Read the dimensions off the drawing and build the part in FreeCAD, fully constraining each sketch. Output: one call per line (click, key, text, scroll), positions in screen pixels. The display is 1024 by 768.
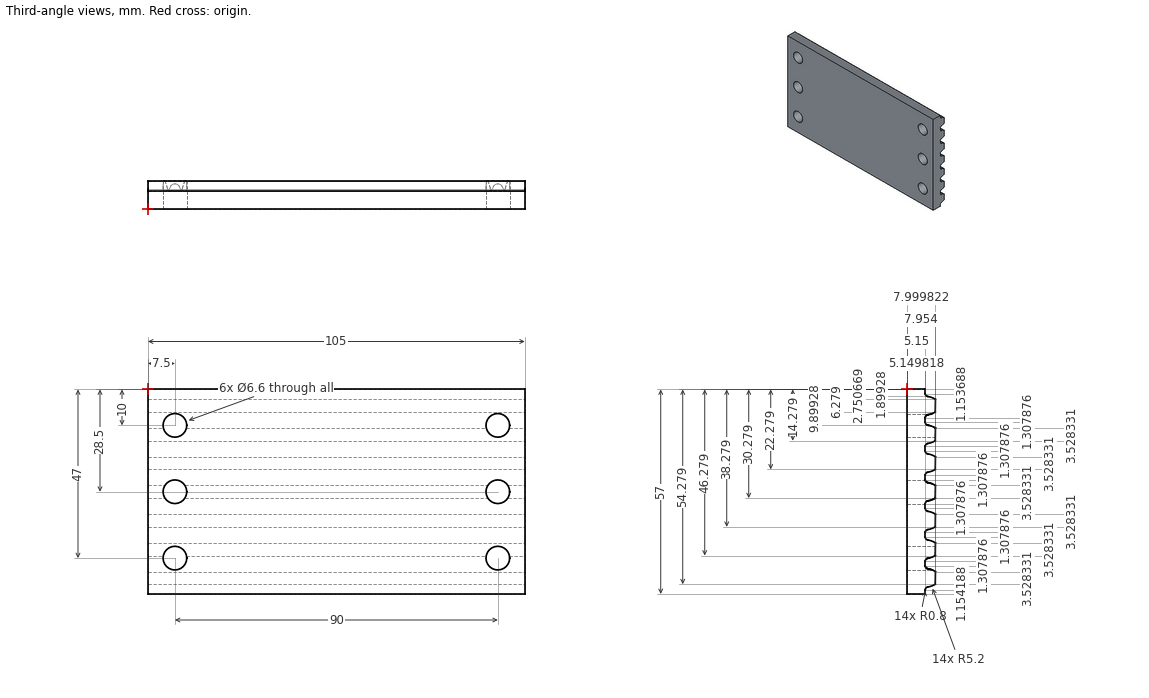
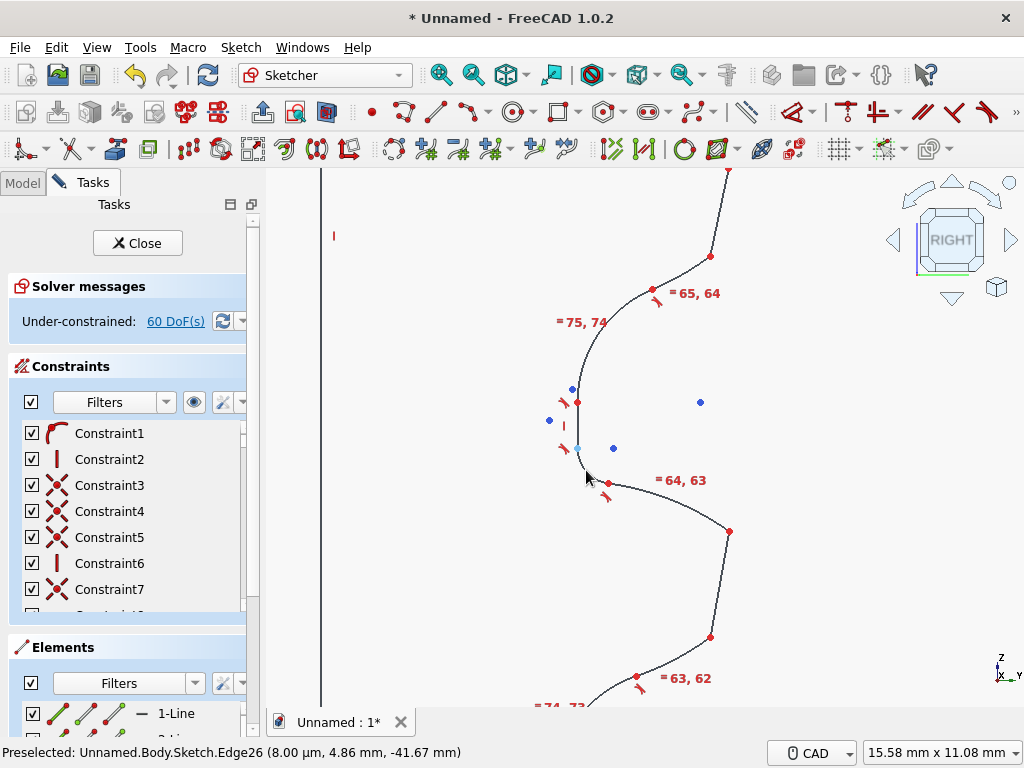
click(581, 463)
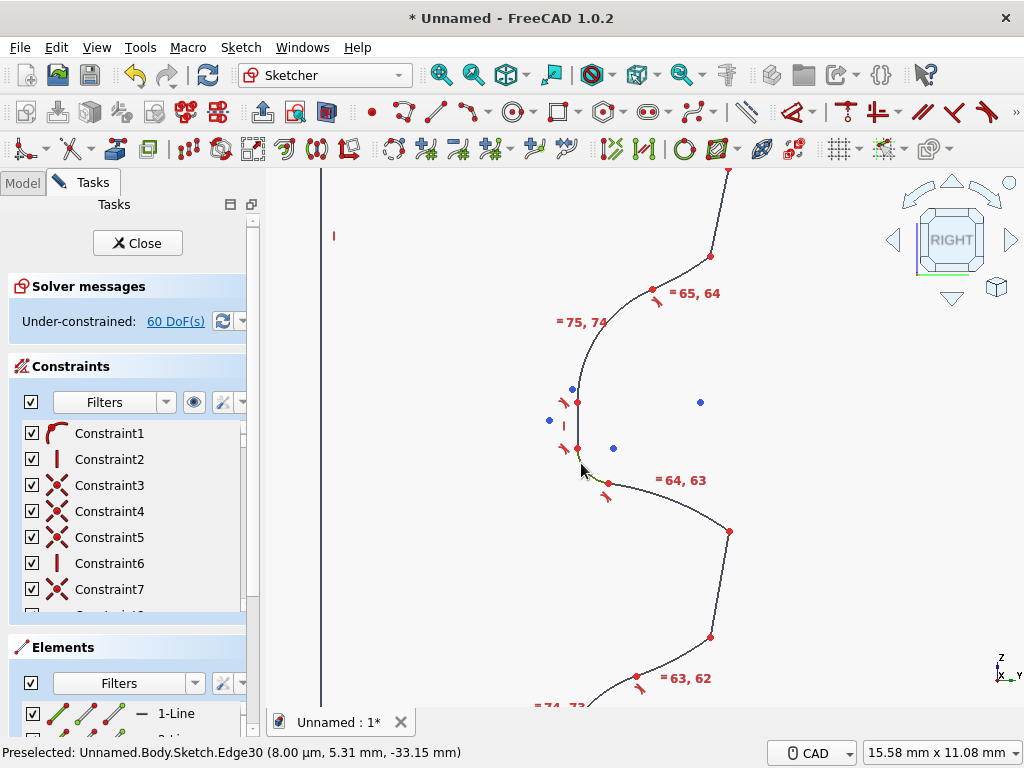
scroll(586, 469, down, 10)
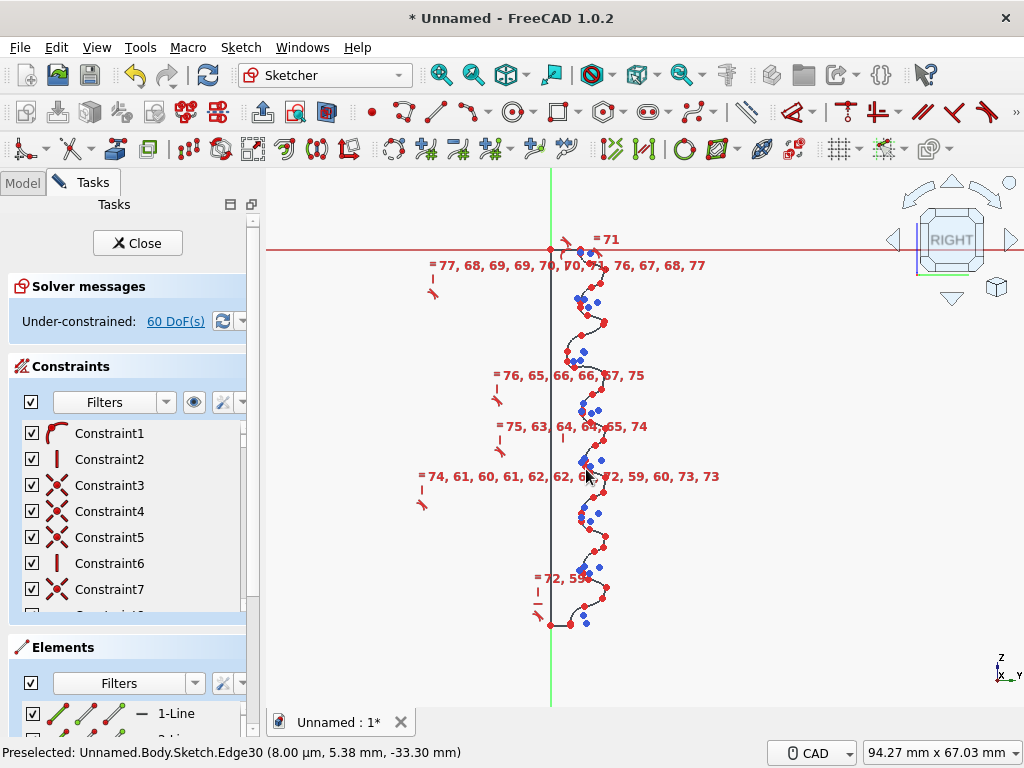
scroll(583, 417, up, 7)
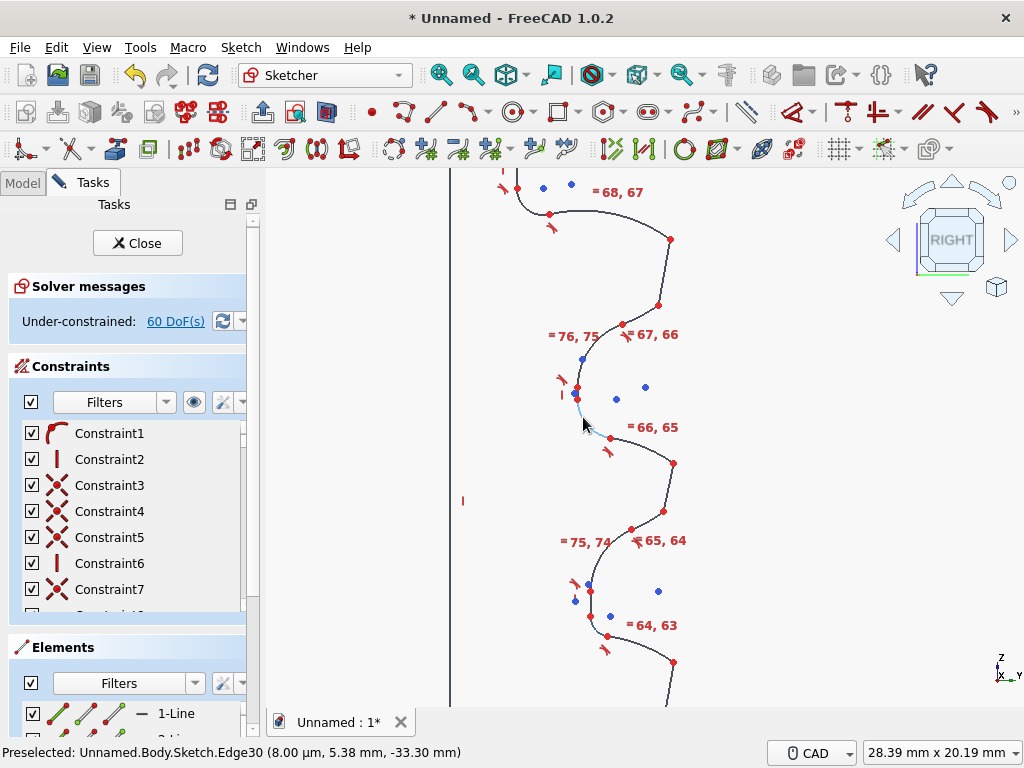
click(581, 416)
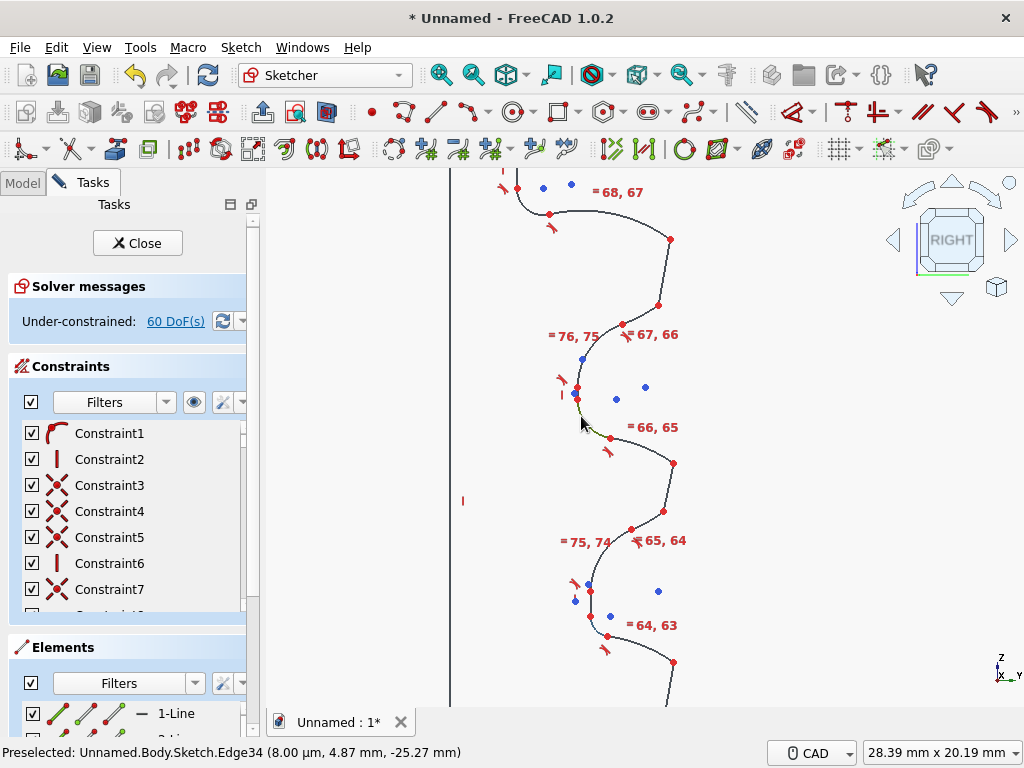
click(521, 202)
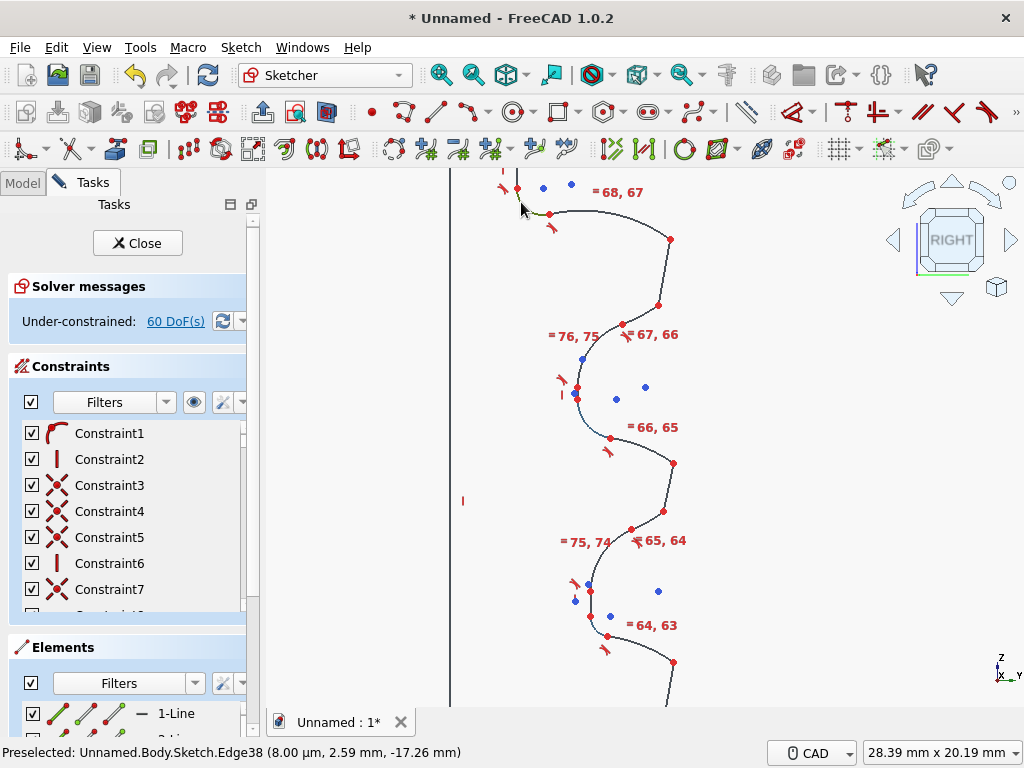
scroll(583, 417, down, 7)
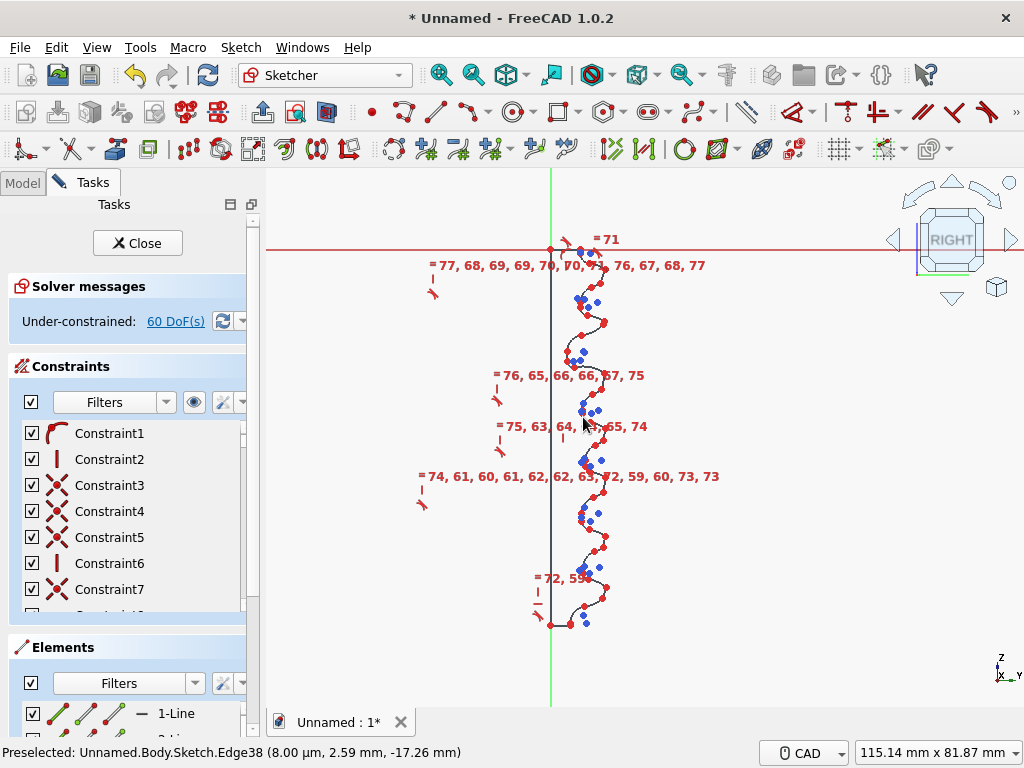
scroll(581, 311, up, 7)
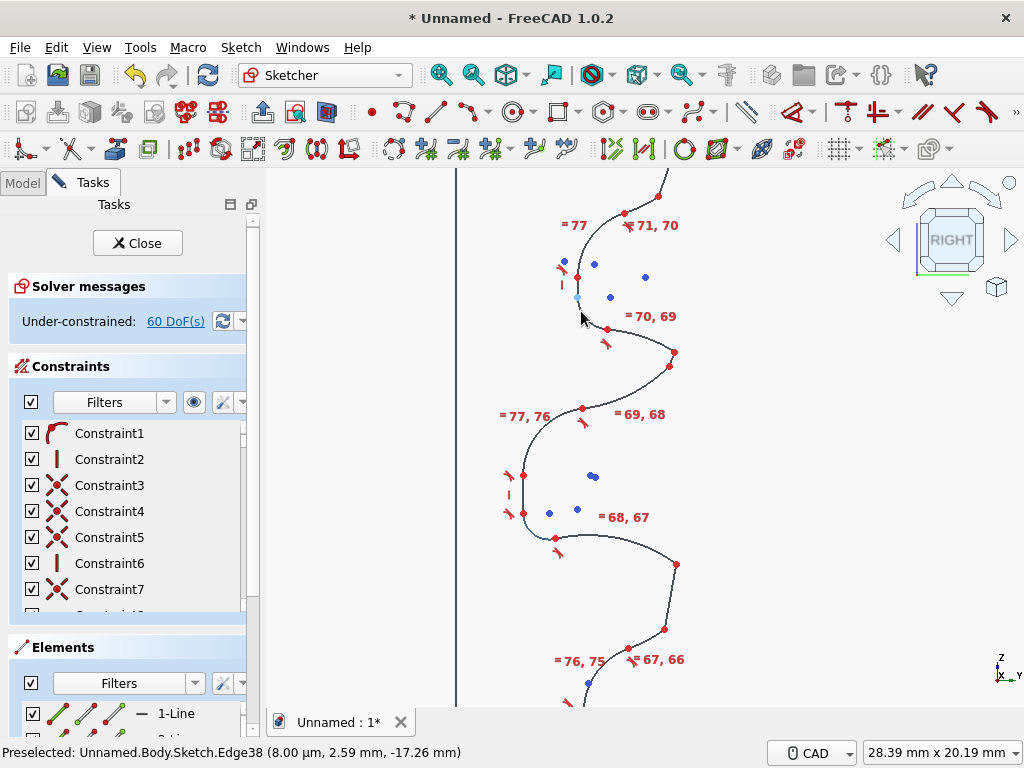
click(581, 311)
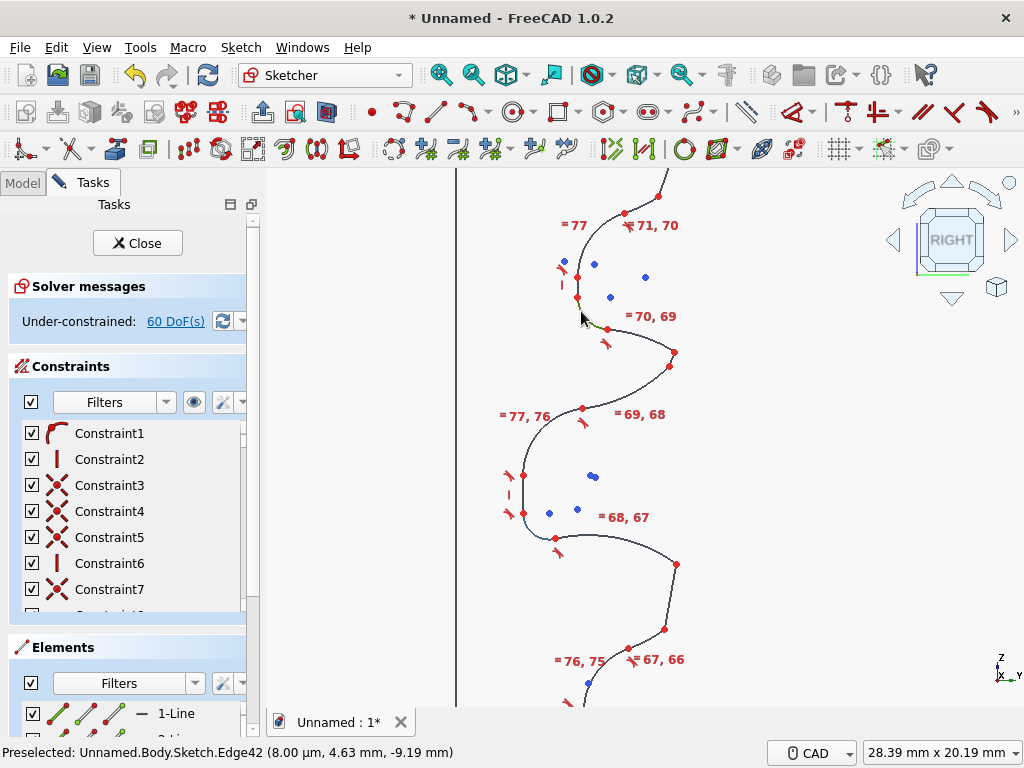
scroll(581, 311, down, 7)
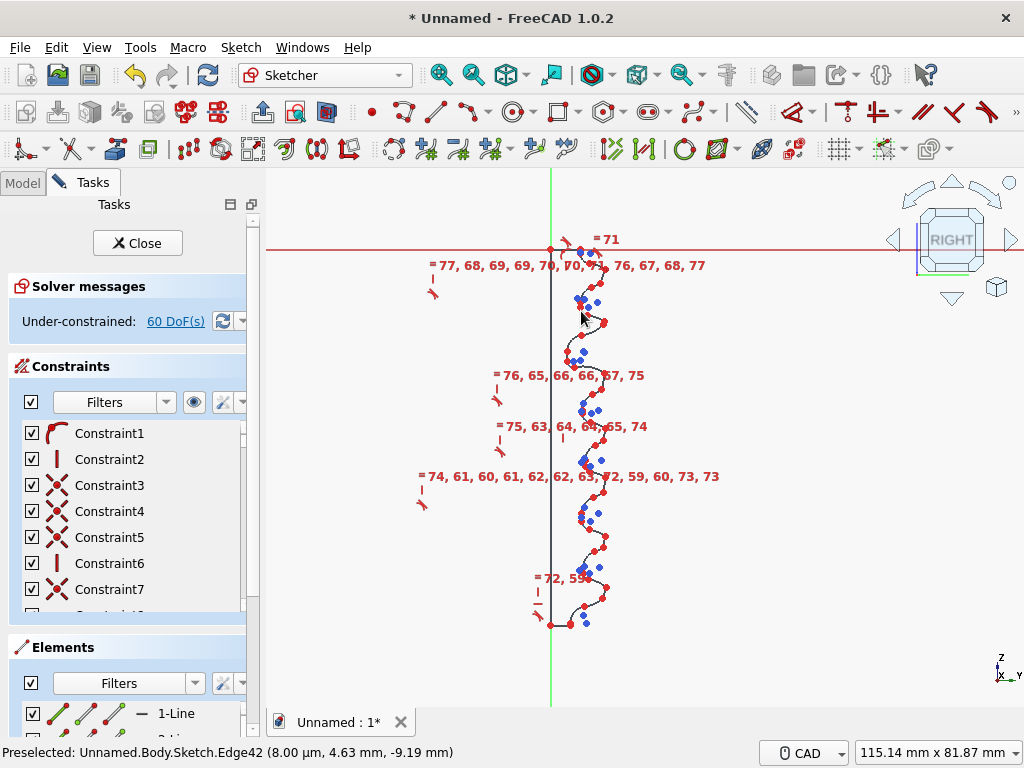
scroll(581, 258, up, 6)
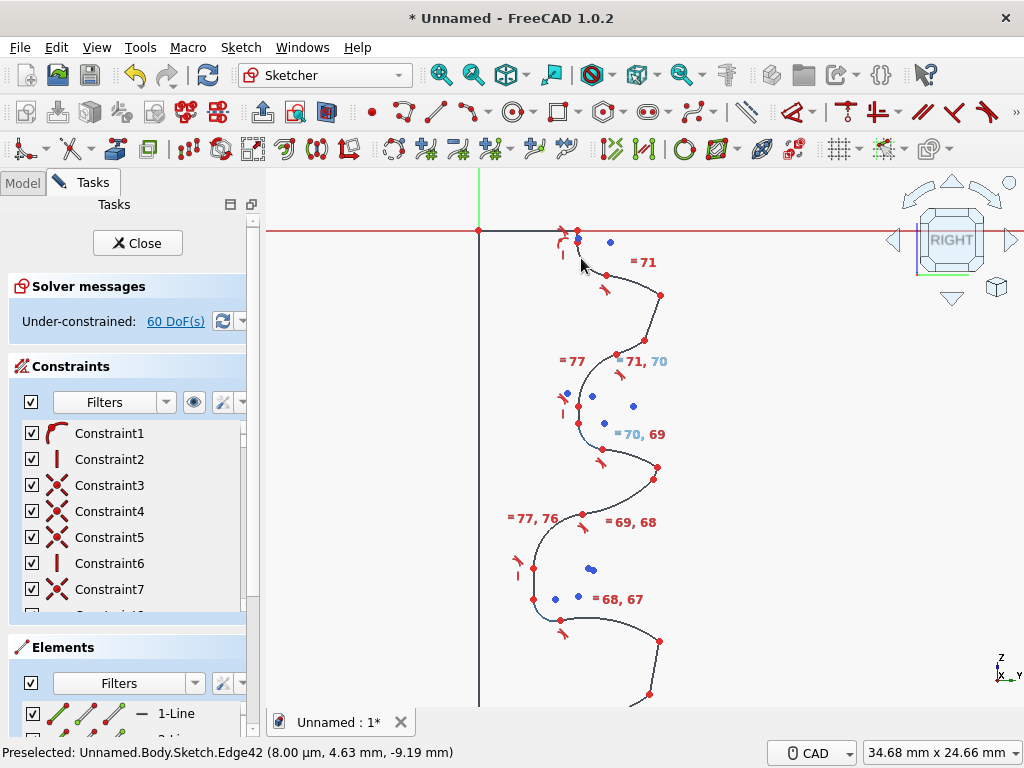
click(580, 256)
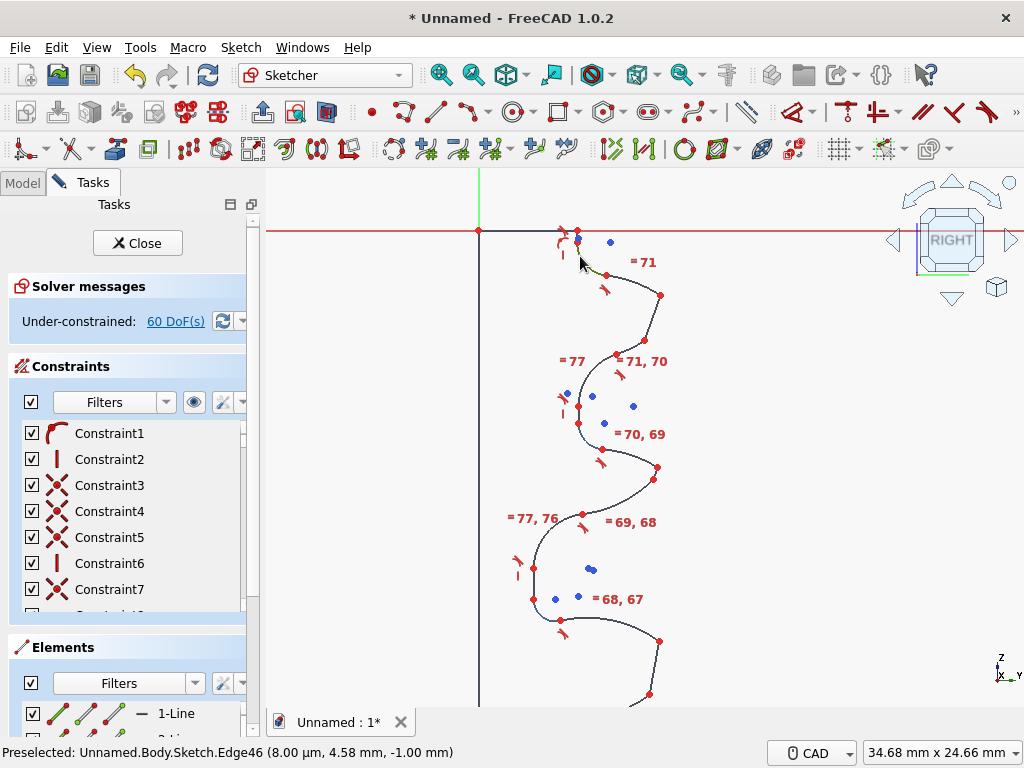
key(e)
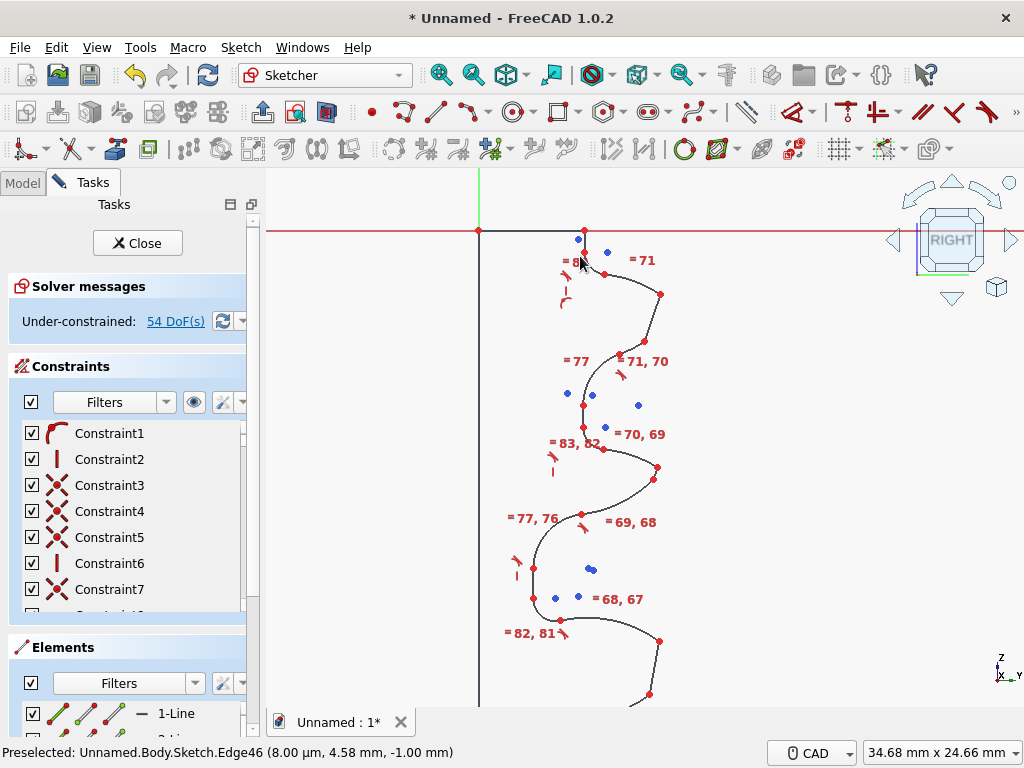
click(792, 112)